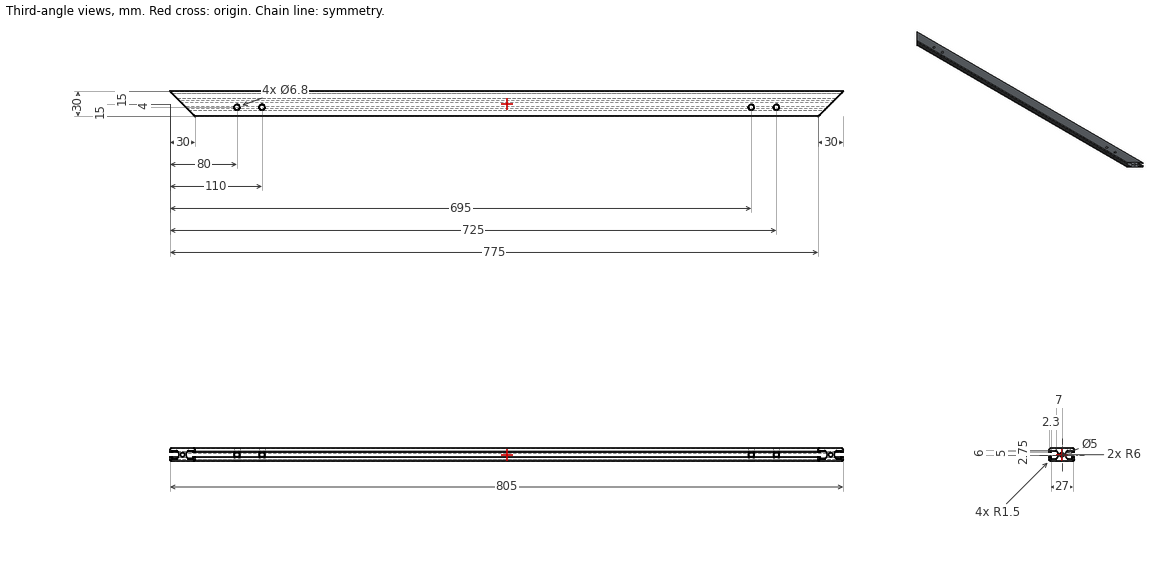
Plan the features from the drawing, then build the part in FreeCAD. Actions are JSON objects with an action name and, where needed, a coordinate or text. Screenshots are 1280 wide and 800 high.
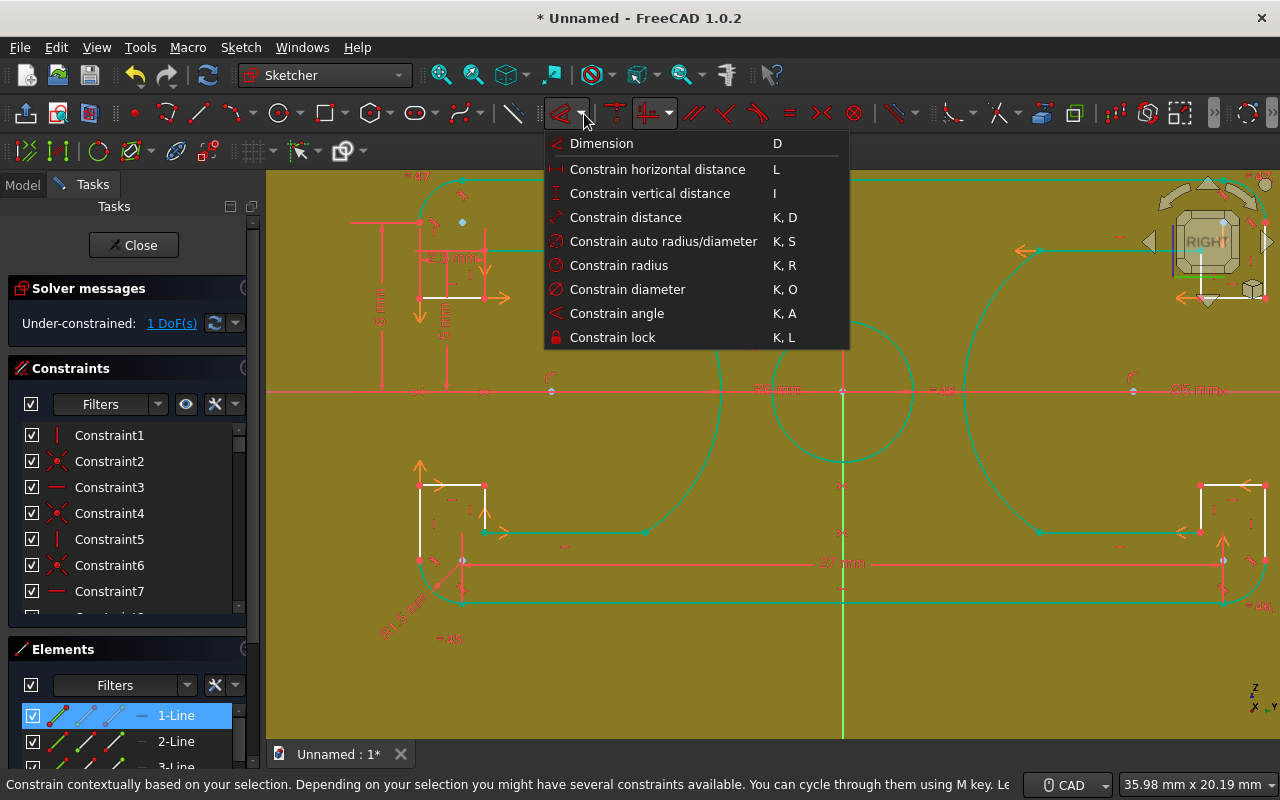
{"action": "left_click", "coordinate": [697, 193]}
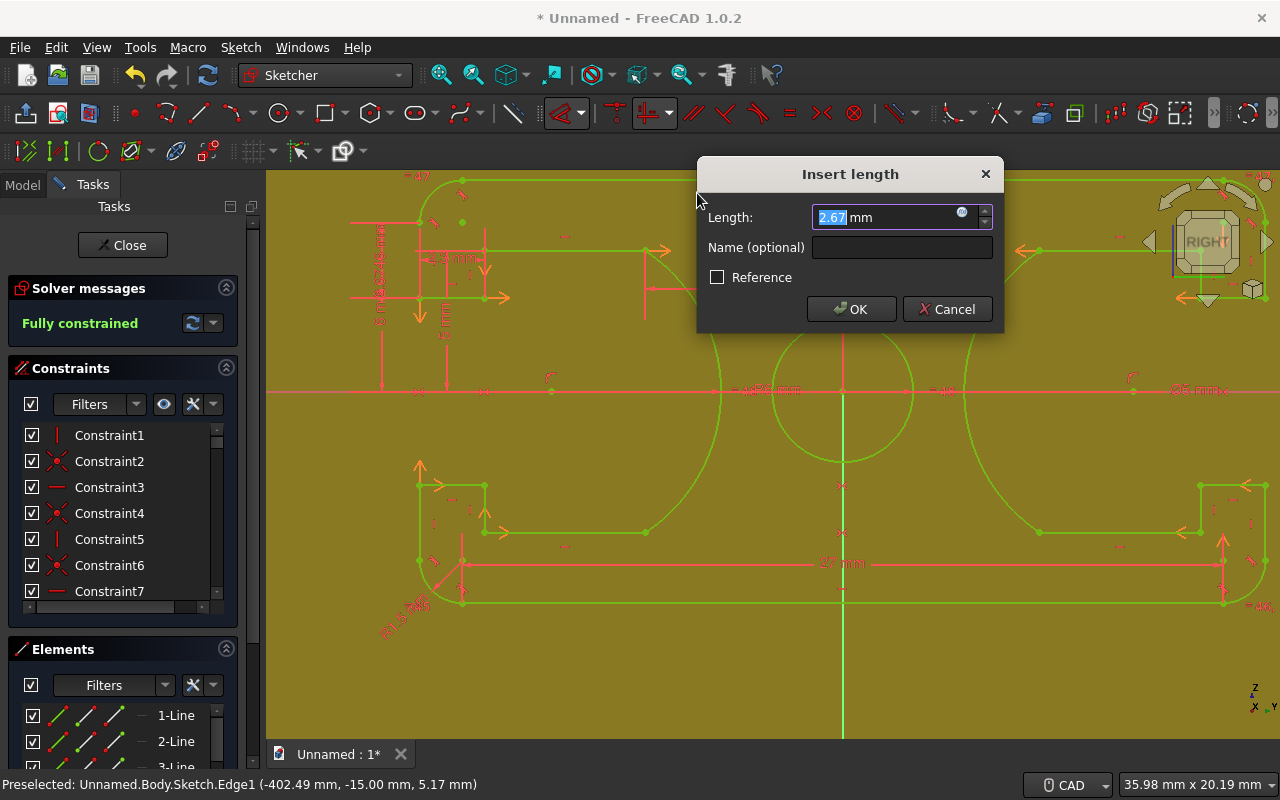
{"action": "type", "text": "2.75"}
{"action": "key", "text": "Return"}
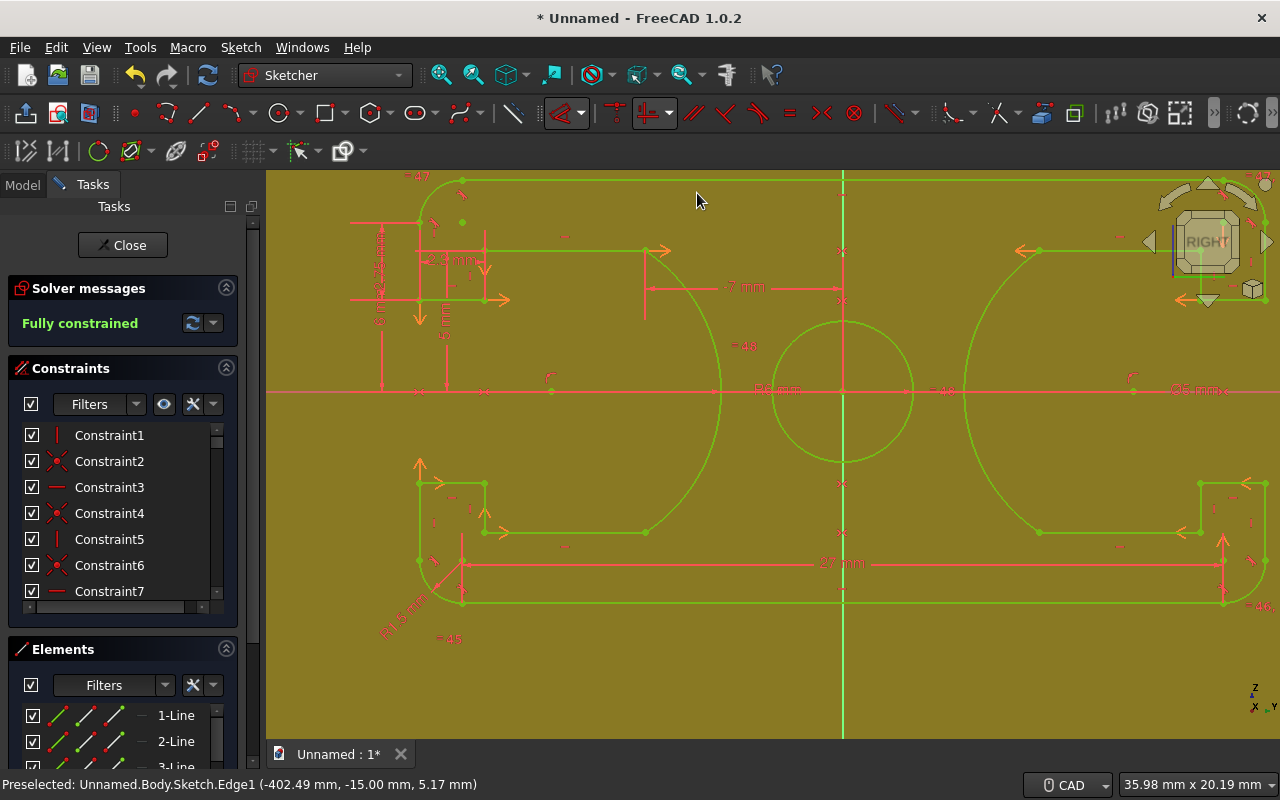
{"action": "left_click", "coordinate": [123, 245]}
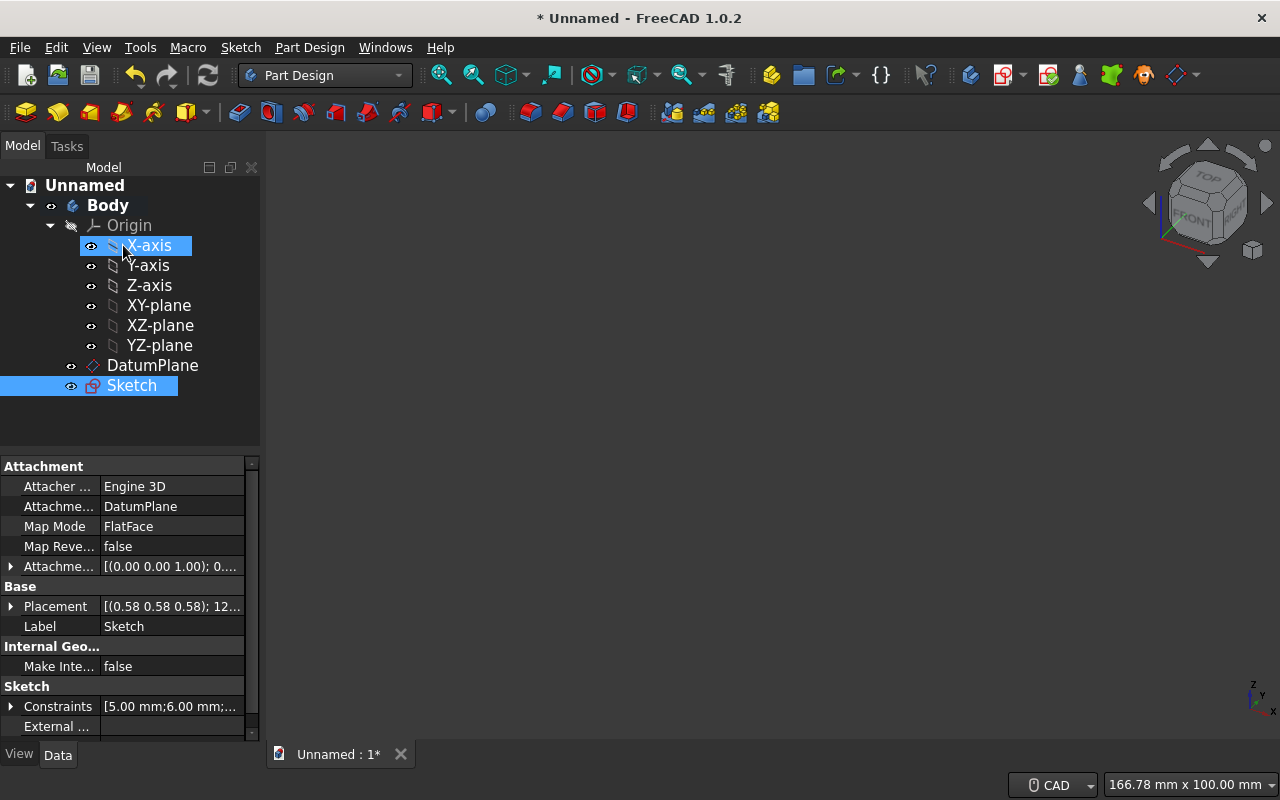
{"action": "left_click", "coordinate": [26, 112]}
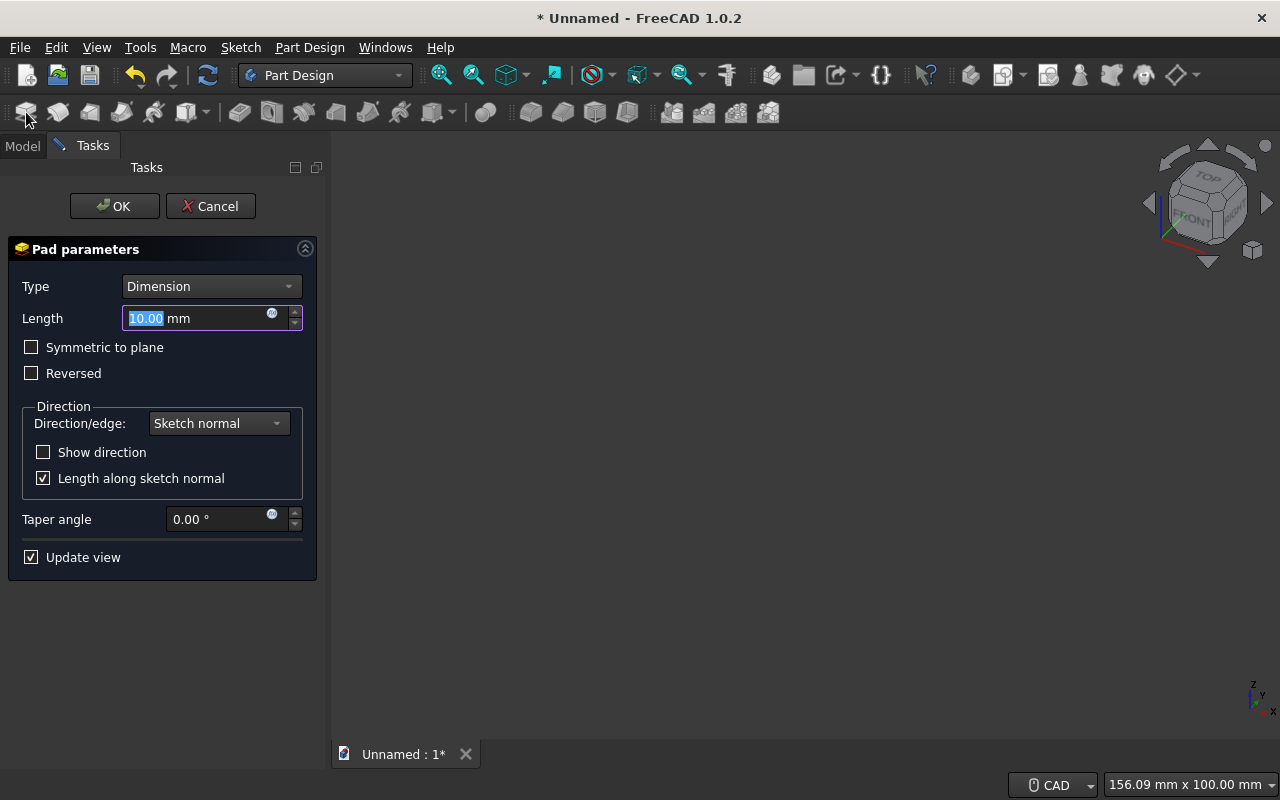
{"action": "type", "text": "805"}
{"action": "key", "text": "Tab"}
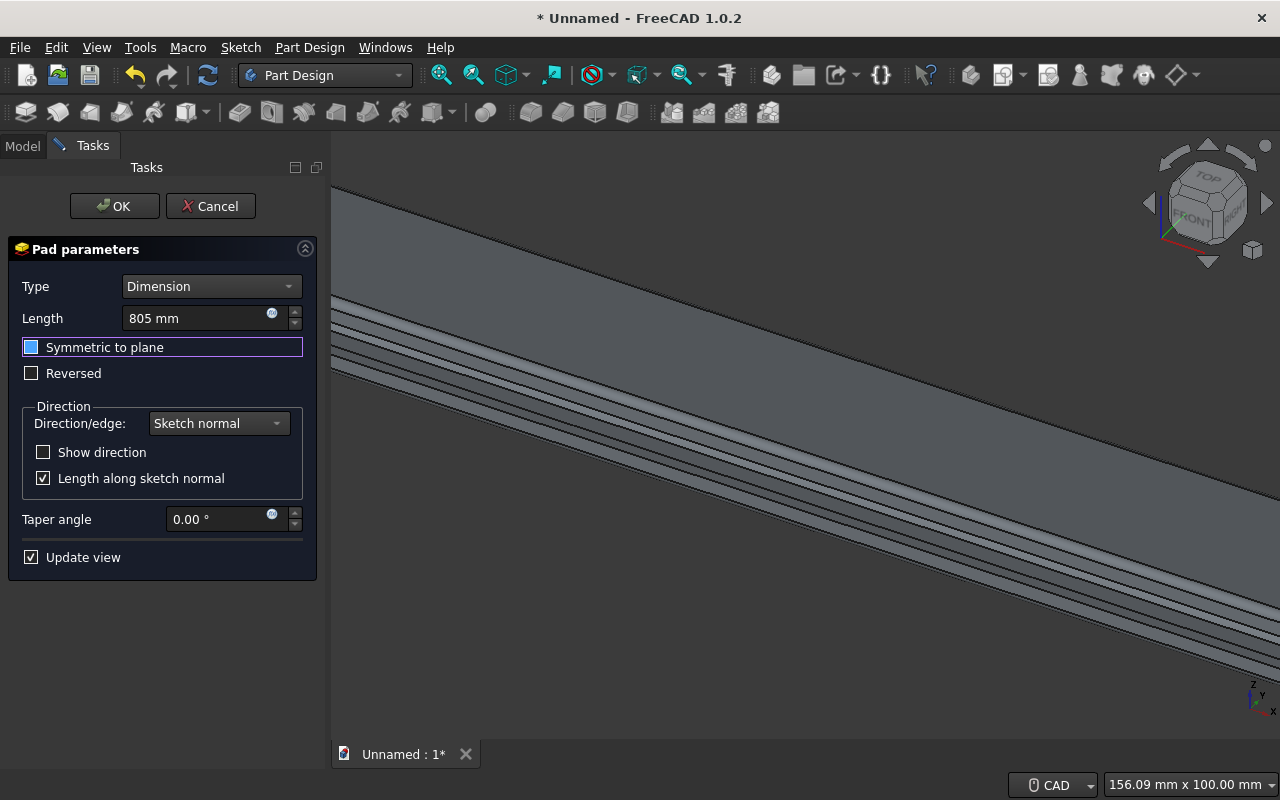
{"action": "left_click", "coordinate": [115, 206]}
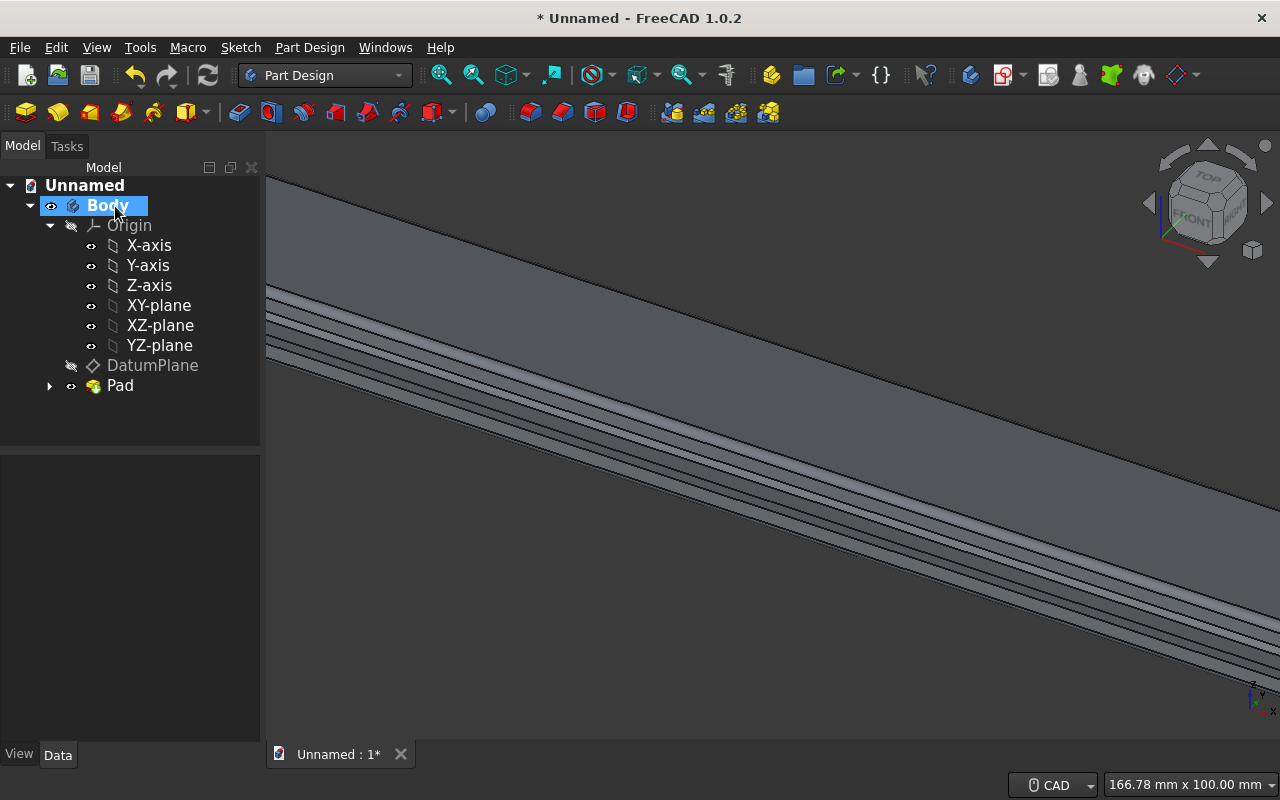
{"action": "left_click", "coordinate": [442, 76]}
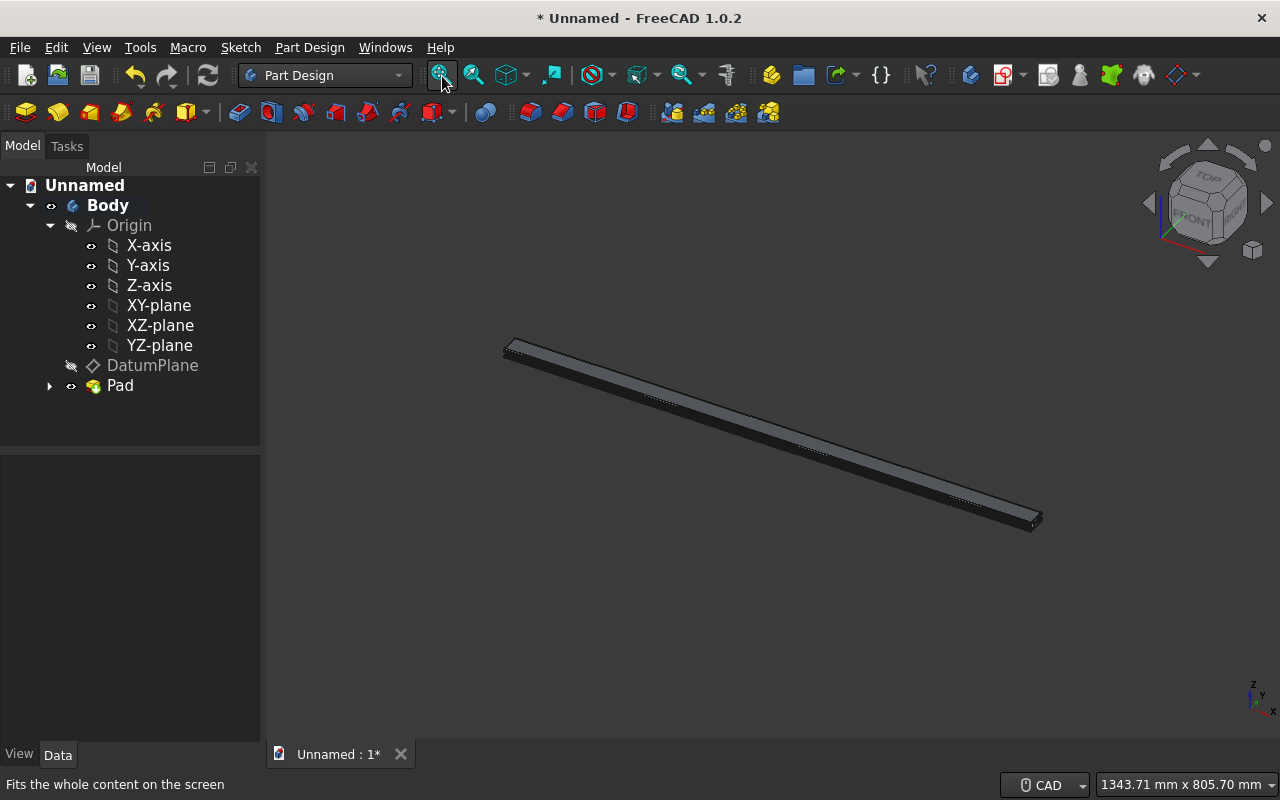
{"action": "key", "text": "0"}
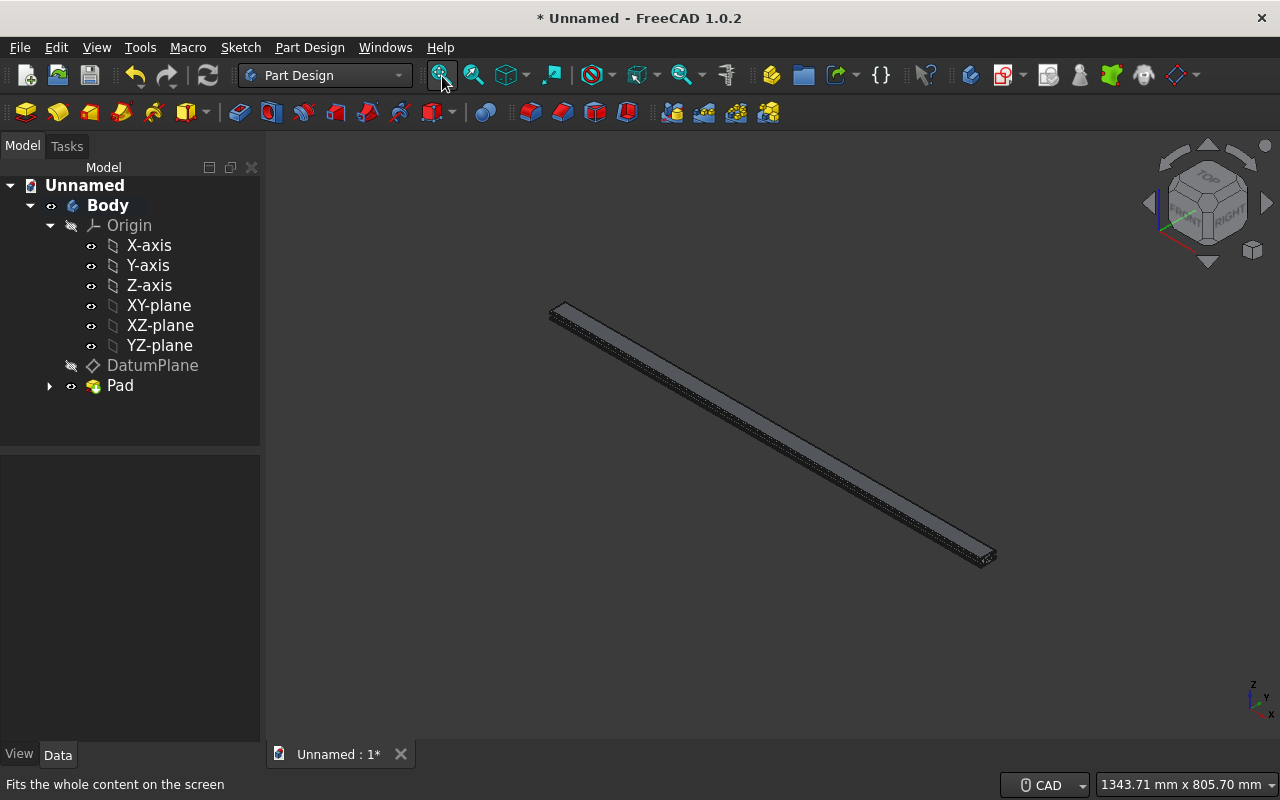
{"action": "left_click", "coordinate": [442, 76]}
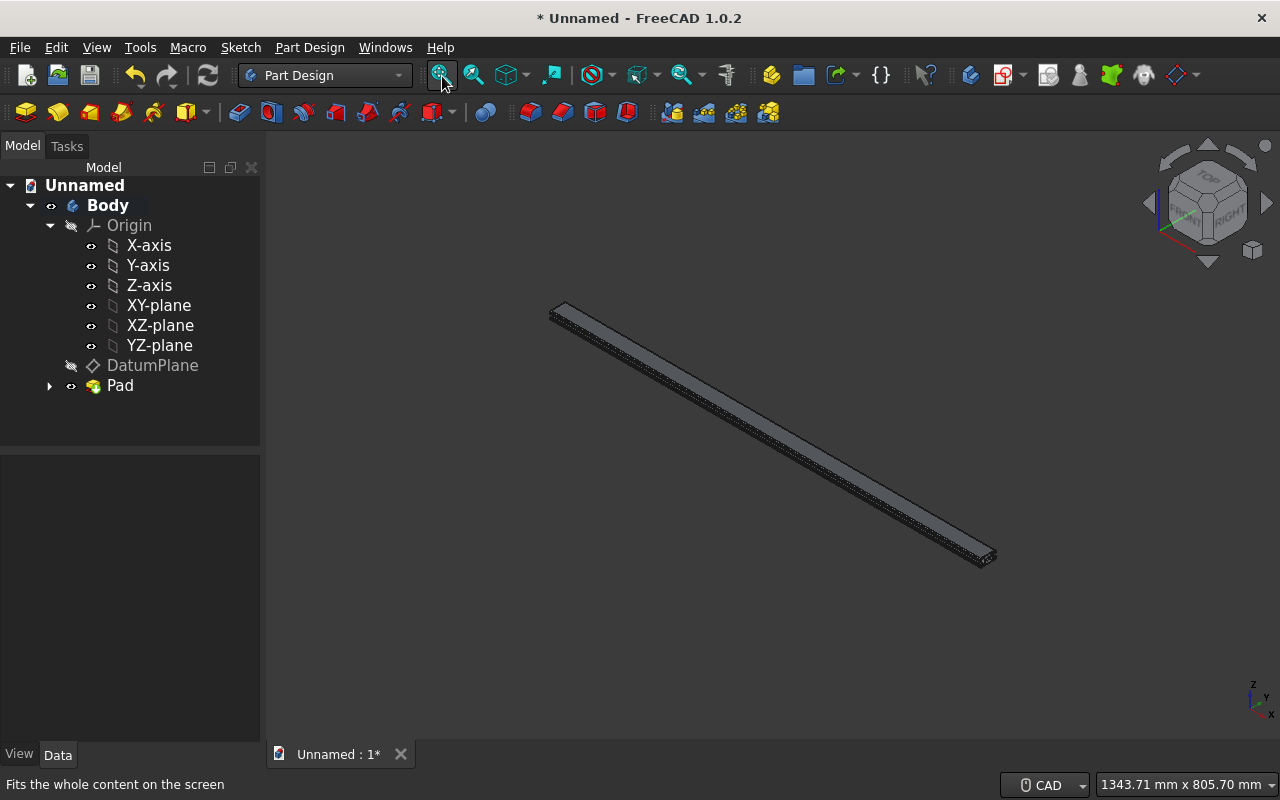
{"action": "key", "text": "2"}